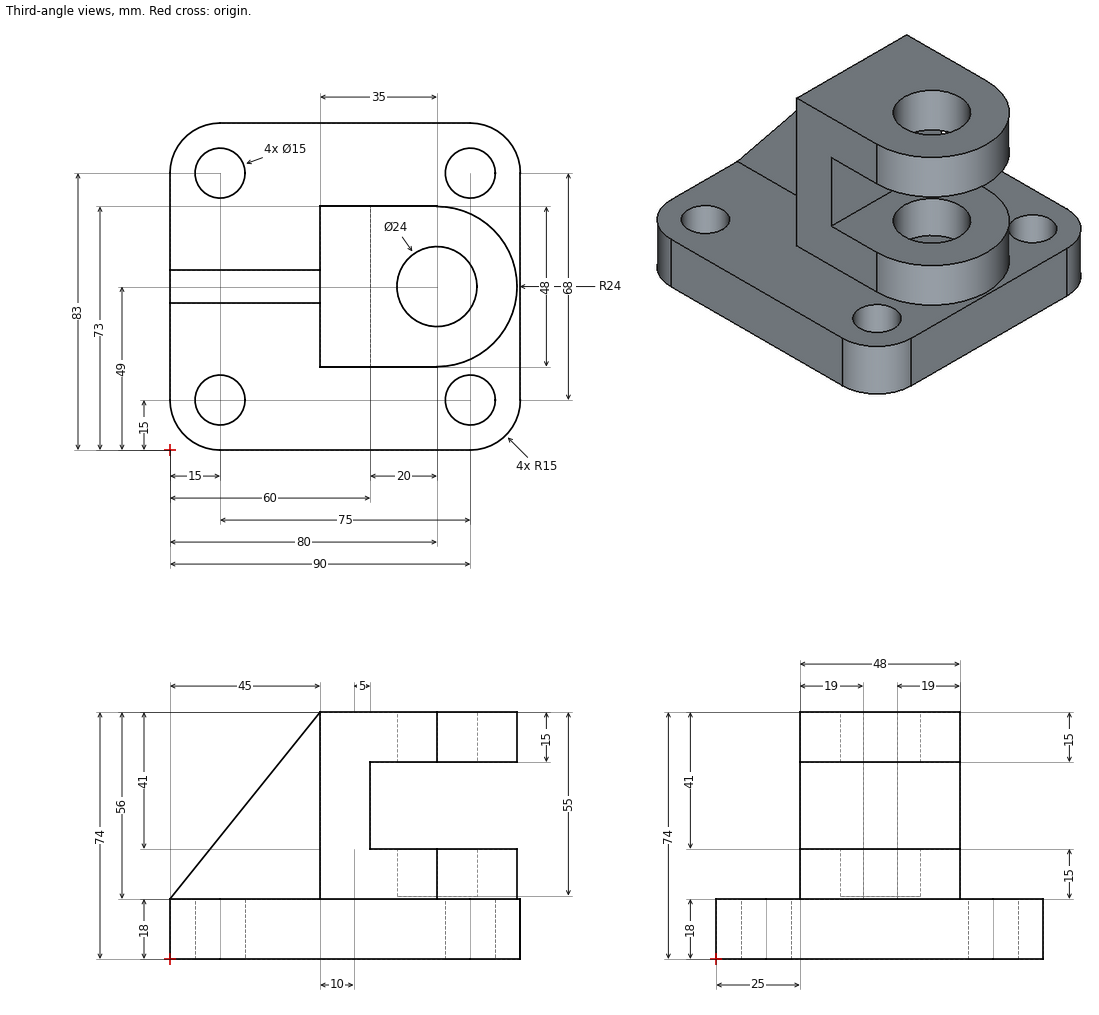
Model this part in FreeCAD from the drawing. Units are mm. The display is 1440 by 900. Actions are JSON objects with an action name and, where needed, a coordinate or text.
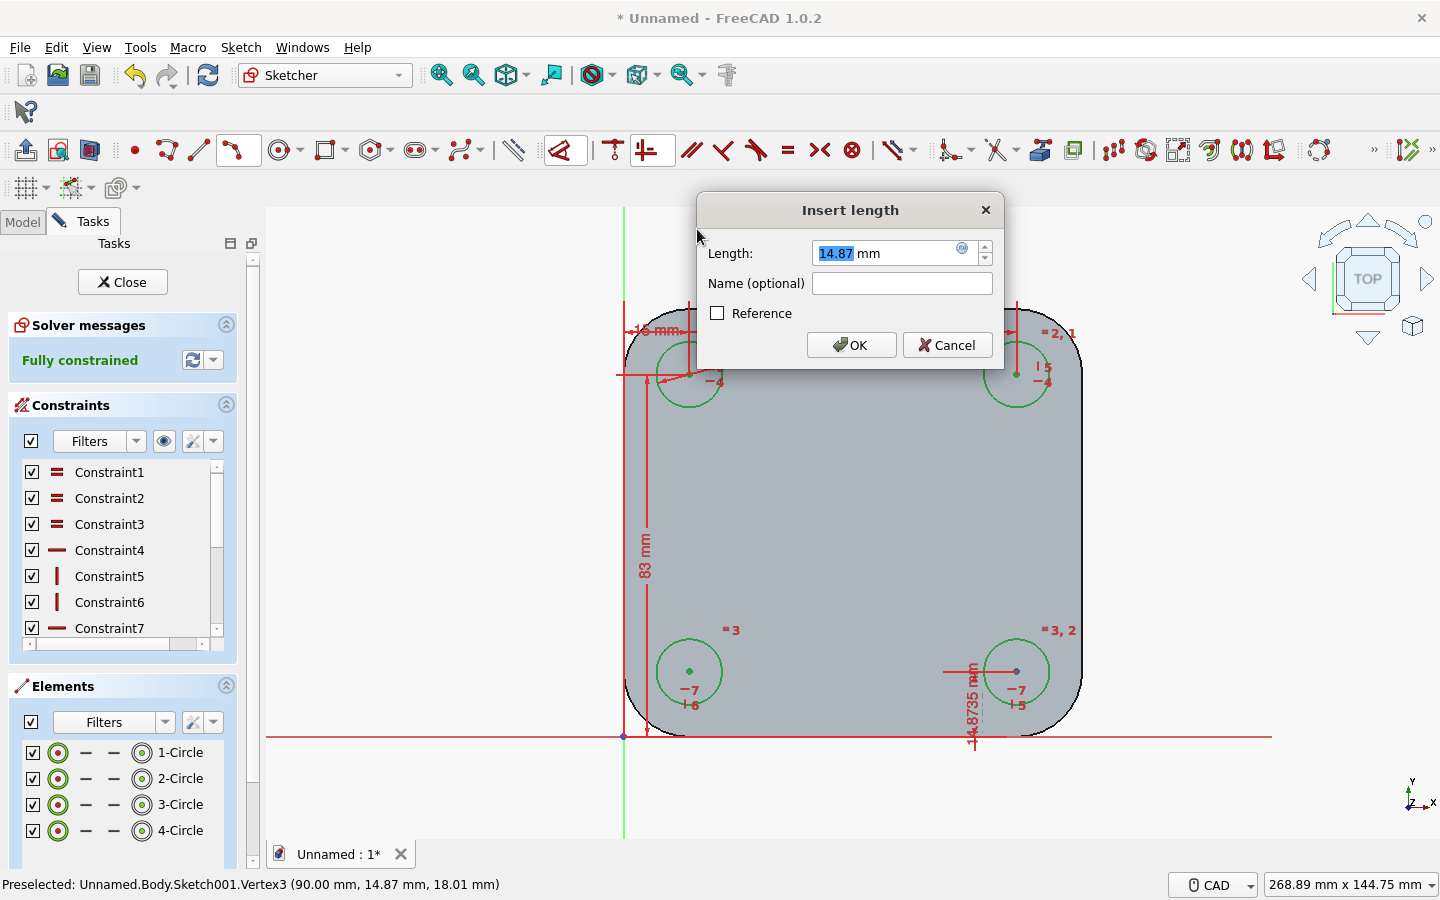
{"action": "type", "text": "15"}
{"action": "key", "text": "Return"}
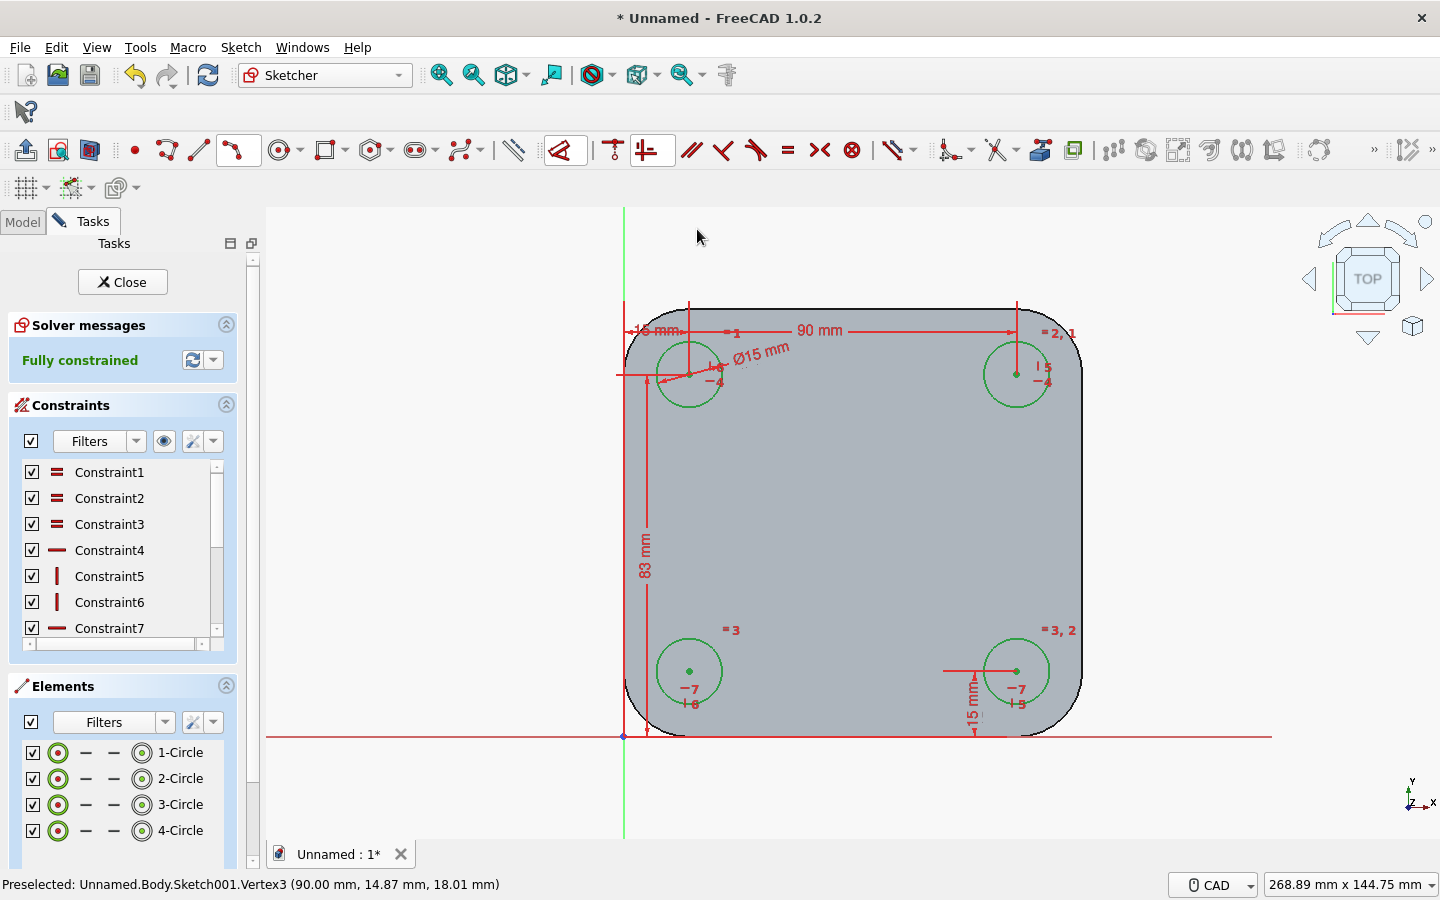
{"action": "left_click", "coordinate": [123, 282]}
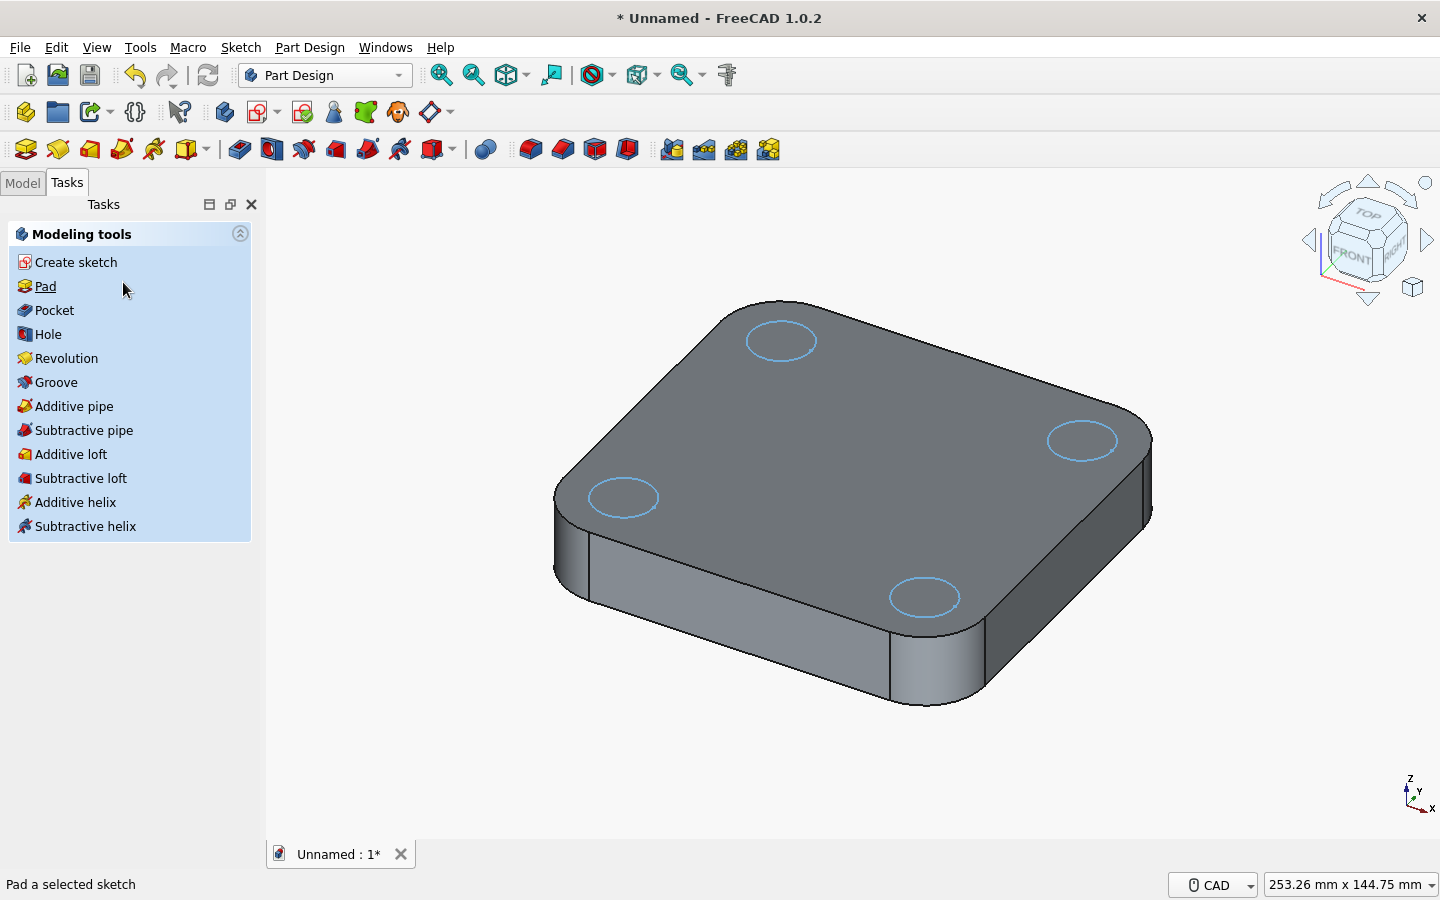
{"action": "left_click", "coordinate": [240, 150]}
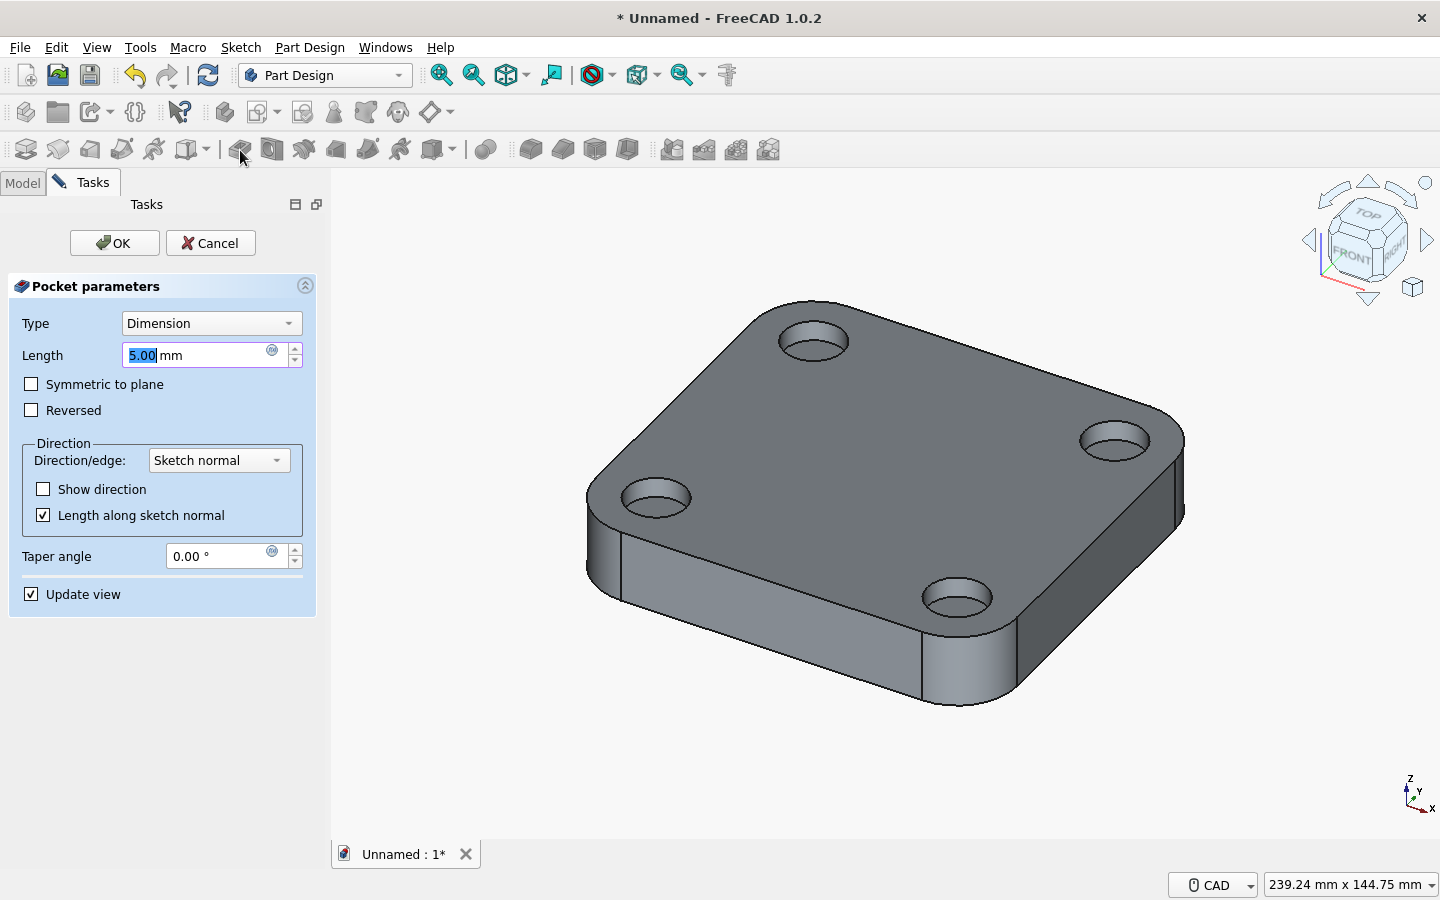
{"action": "type", "text": "18"}
{"action": "key", "text": "Tab"}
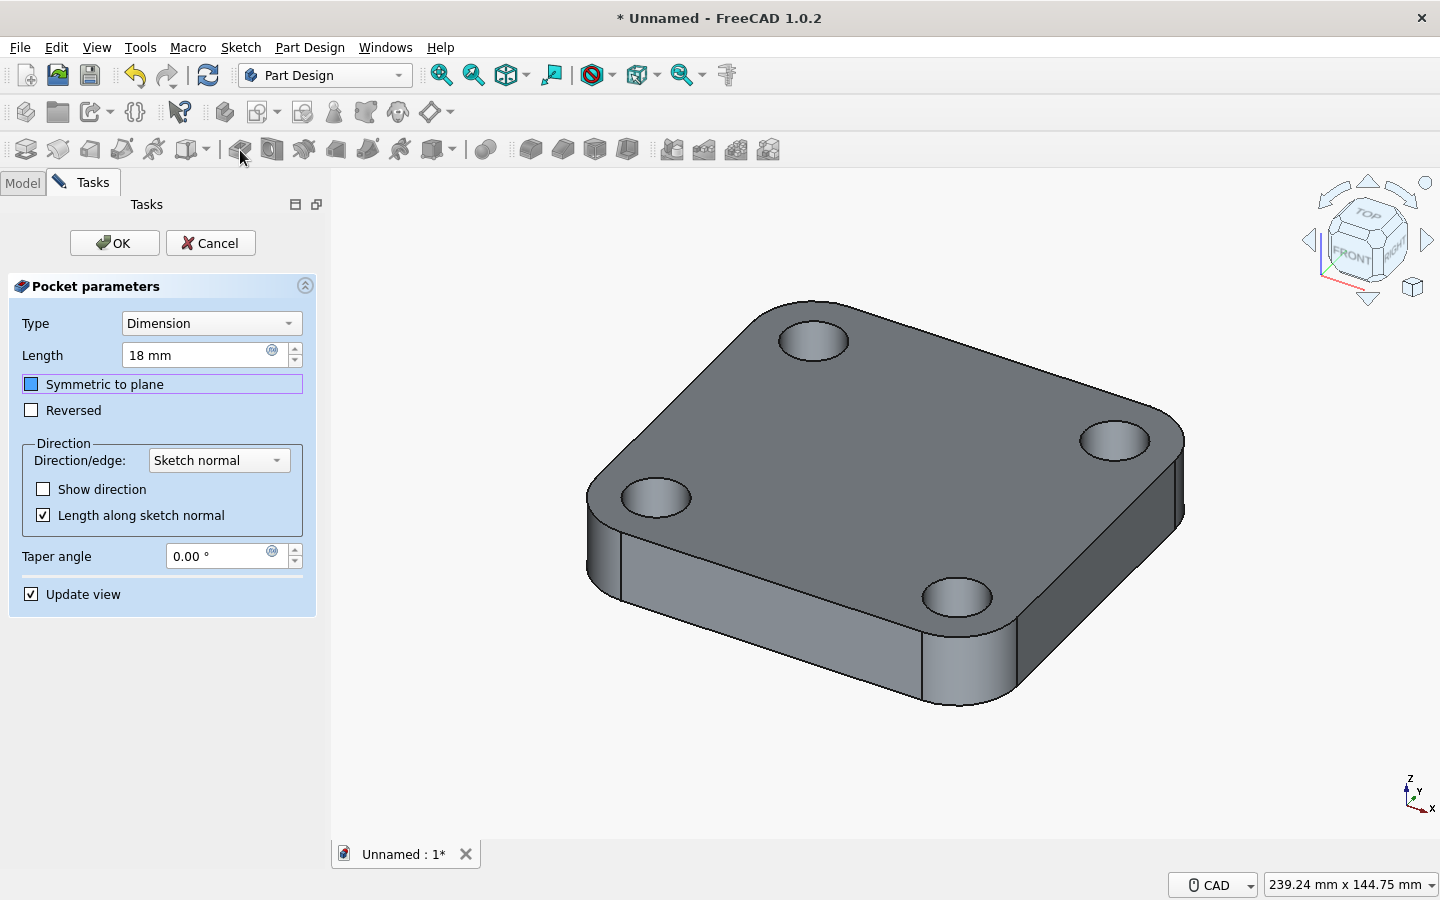
{"action": "left_click", "coordinate": [115, 243]}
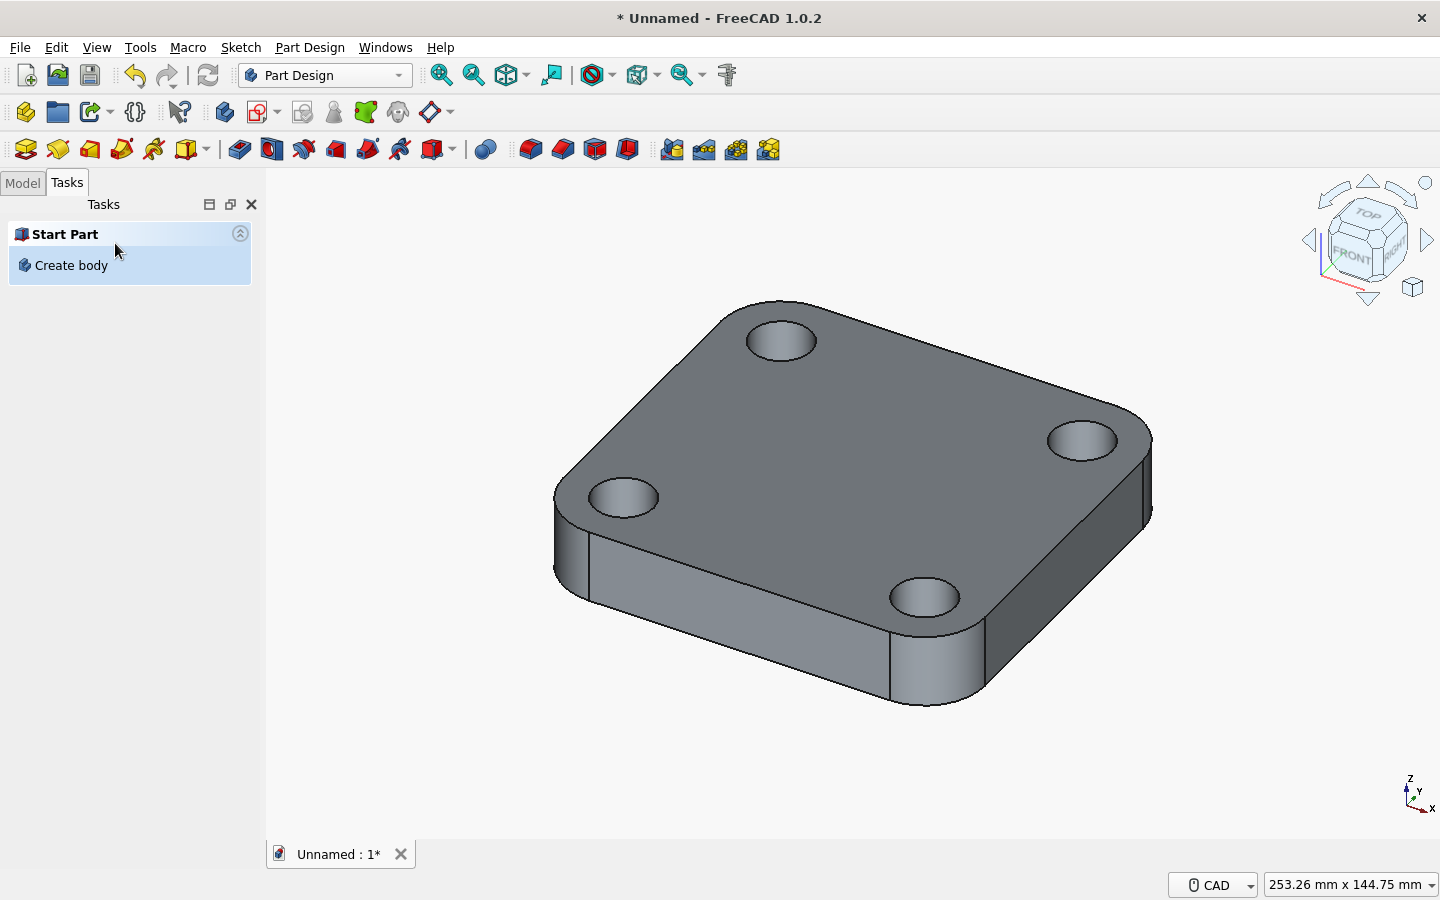
{"action": "left_click", "coordinate": [853, 468]}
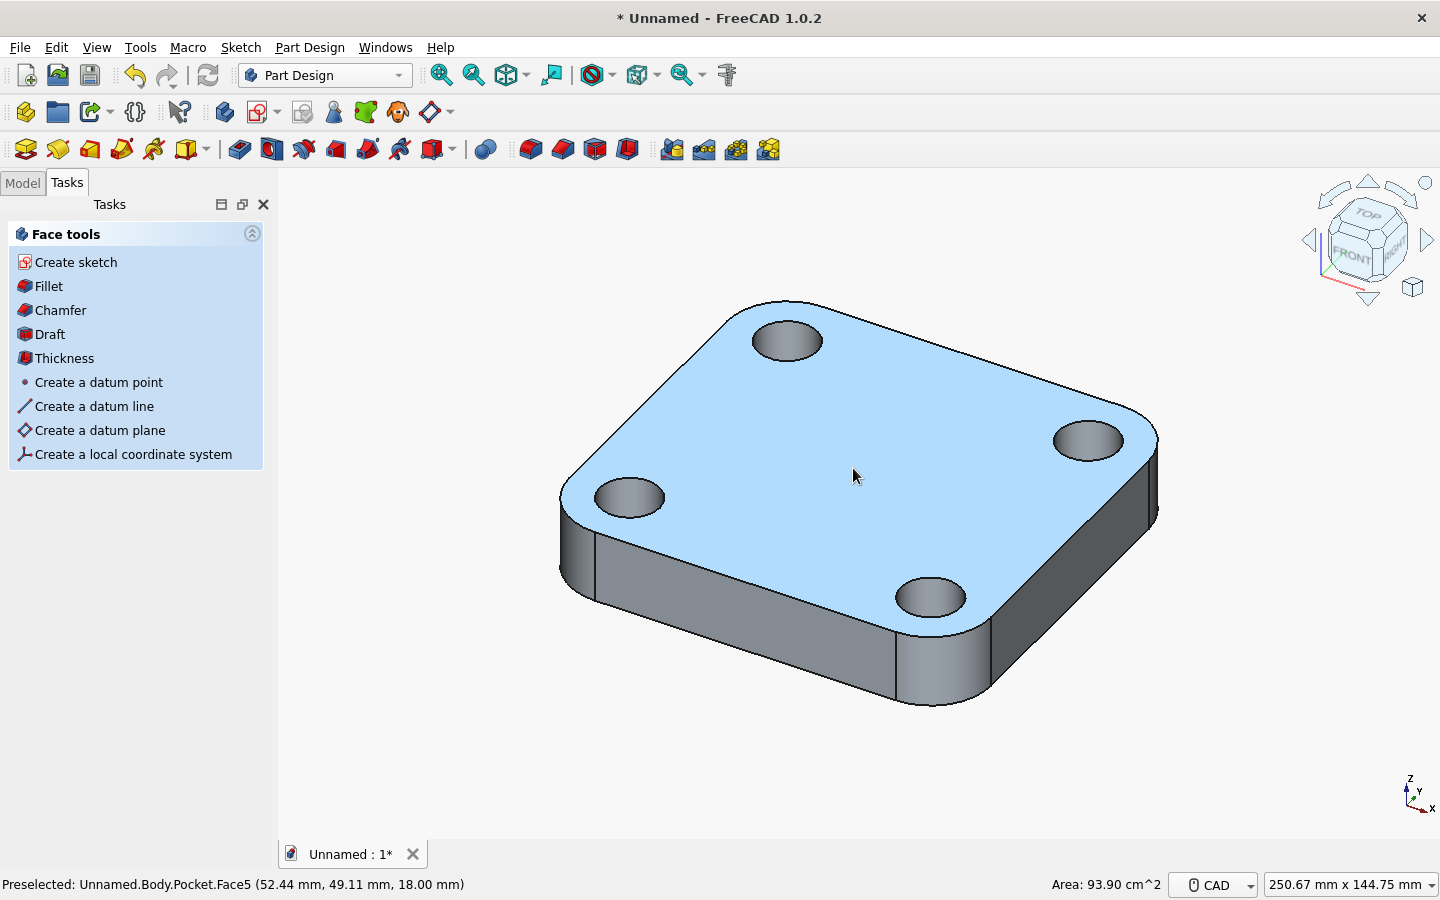
{"action": "left_click", "coordinate": [258, 112]}